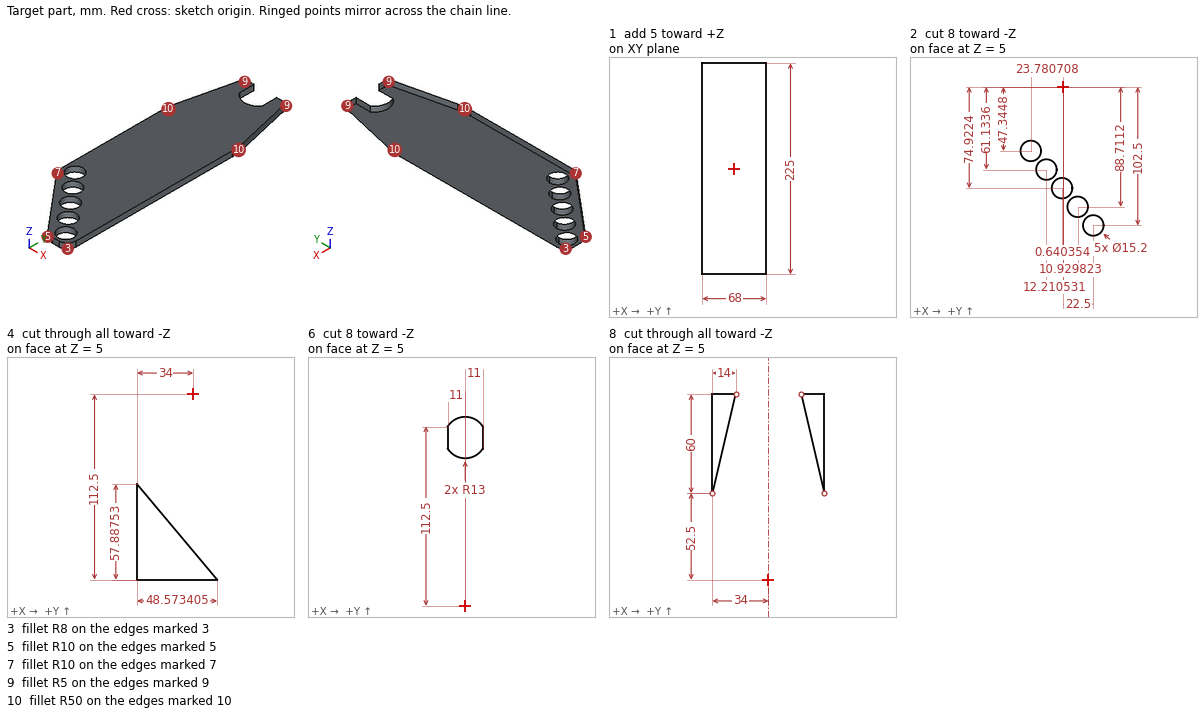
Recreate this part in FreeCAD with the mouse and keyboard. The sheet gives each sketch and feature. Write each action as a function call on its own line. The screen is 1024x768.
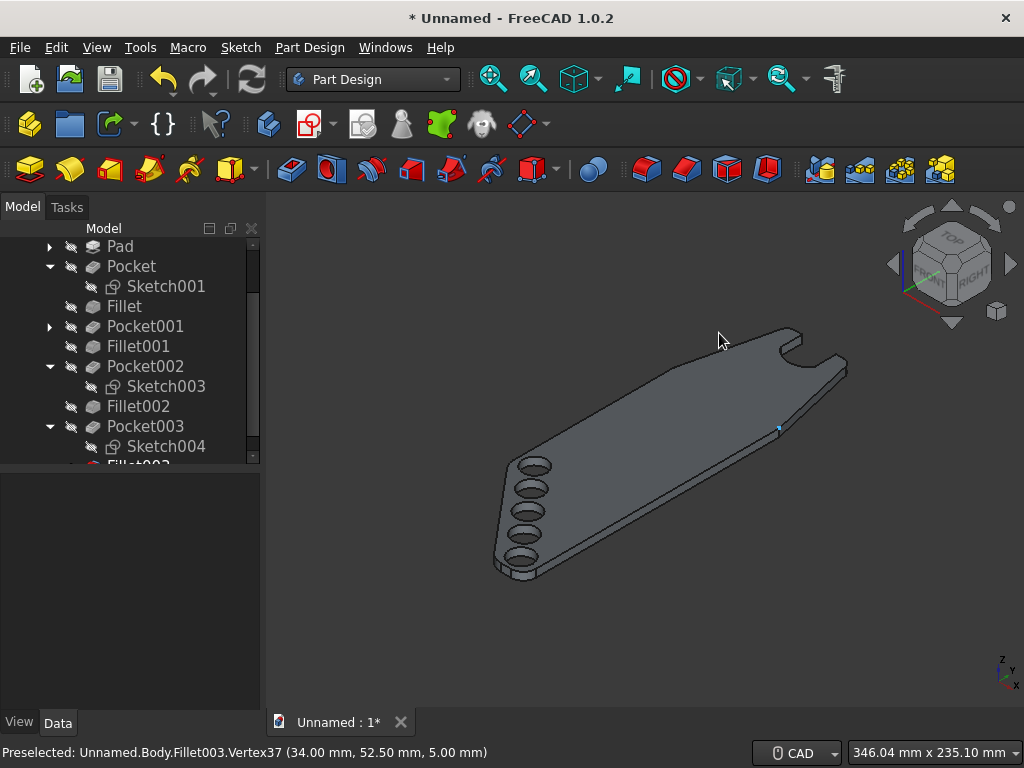
scroll(779, 432, up, 7)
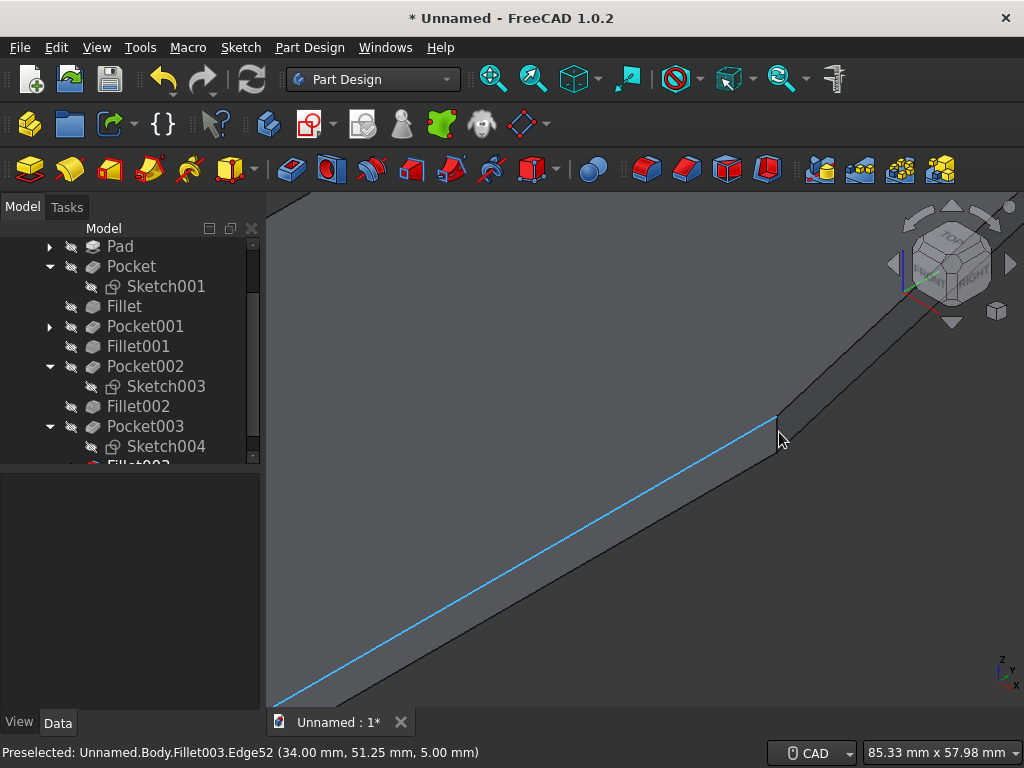
key(v)
key(f)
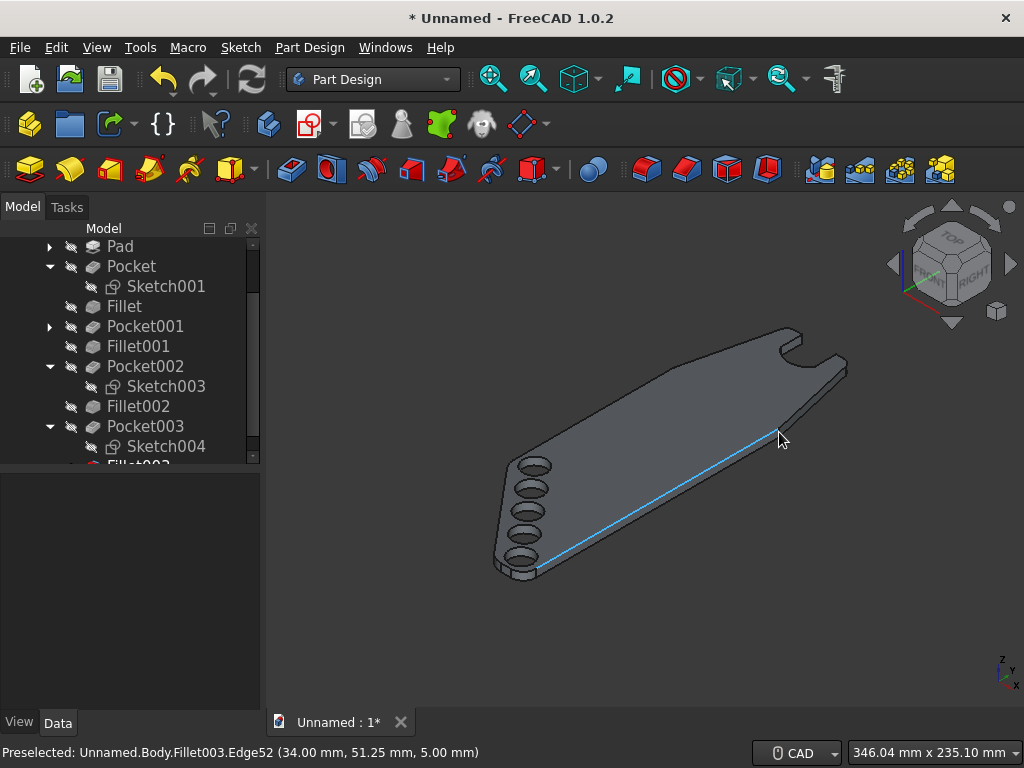
key(1)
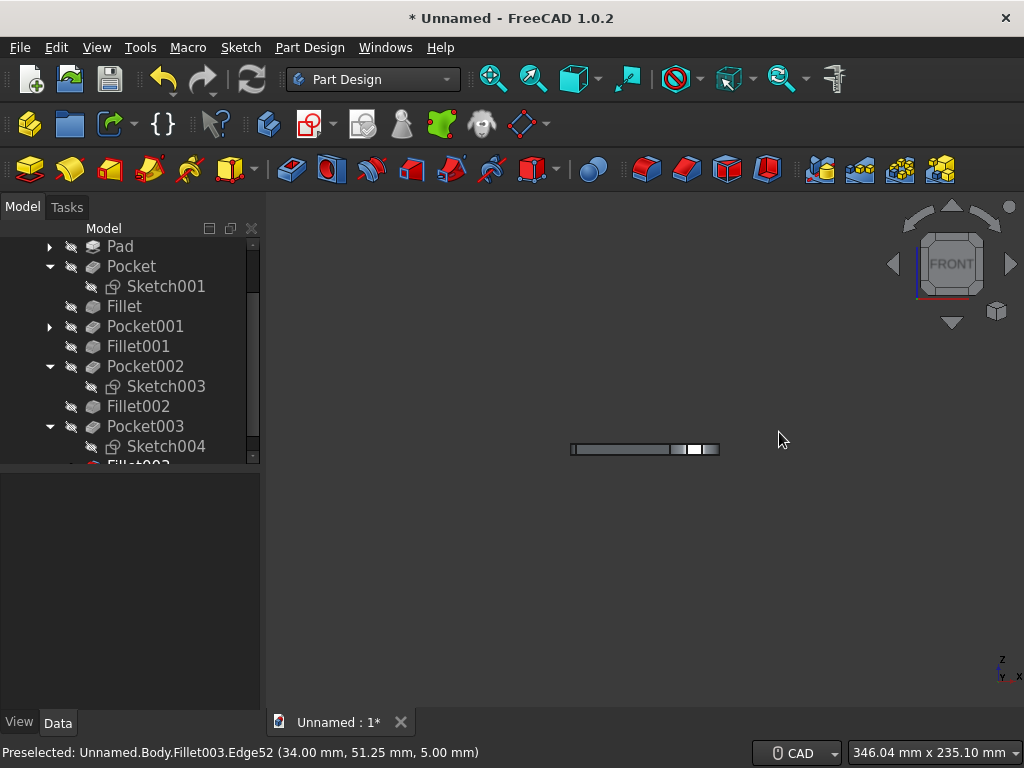
click(494, 80)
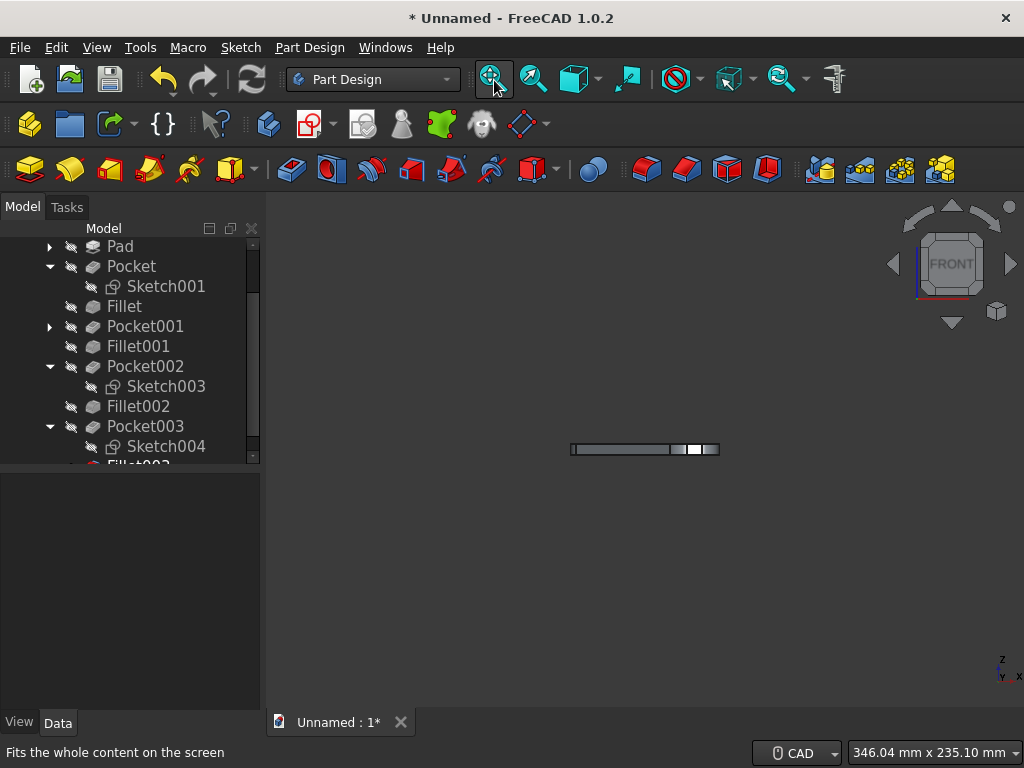
scroll(719, 449, up, 7)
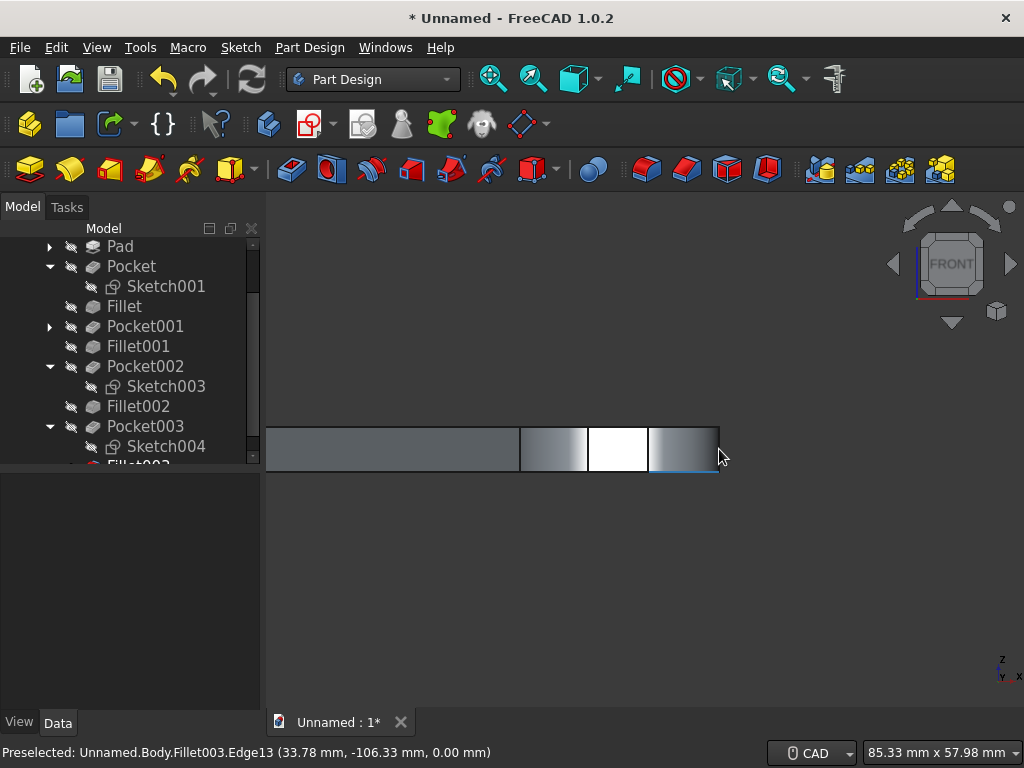
key(v)
key(f)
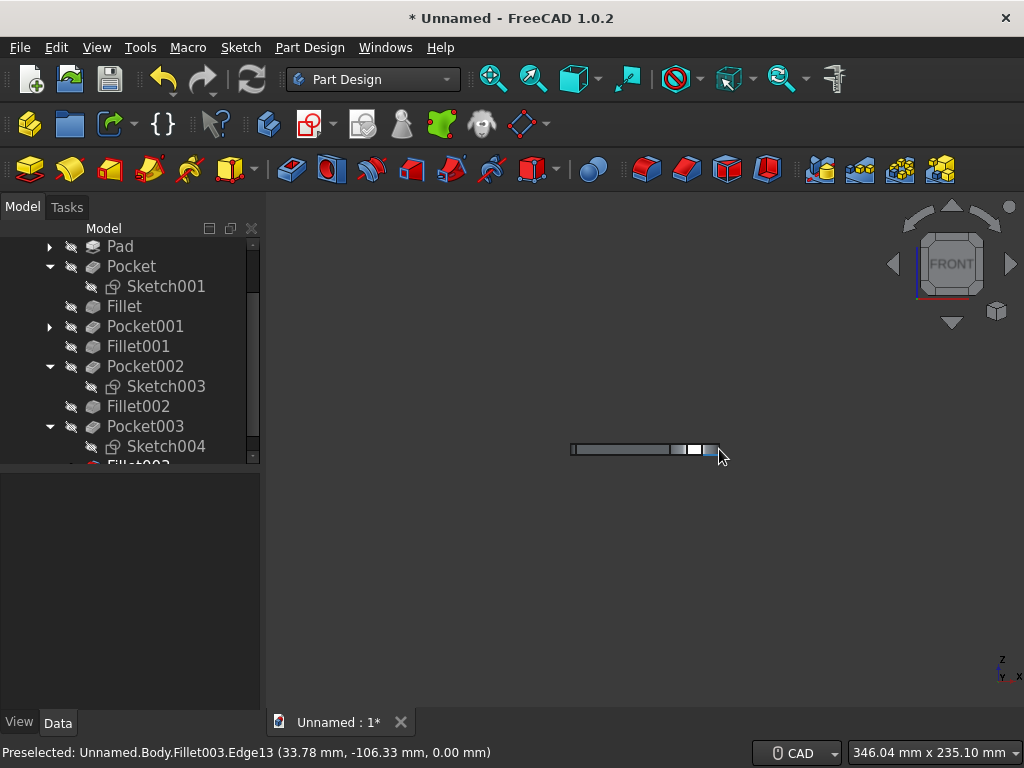
key(3)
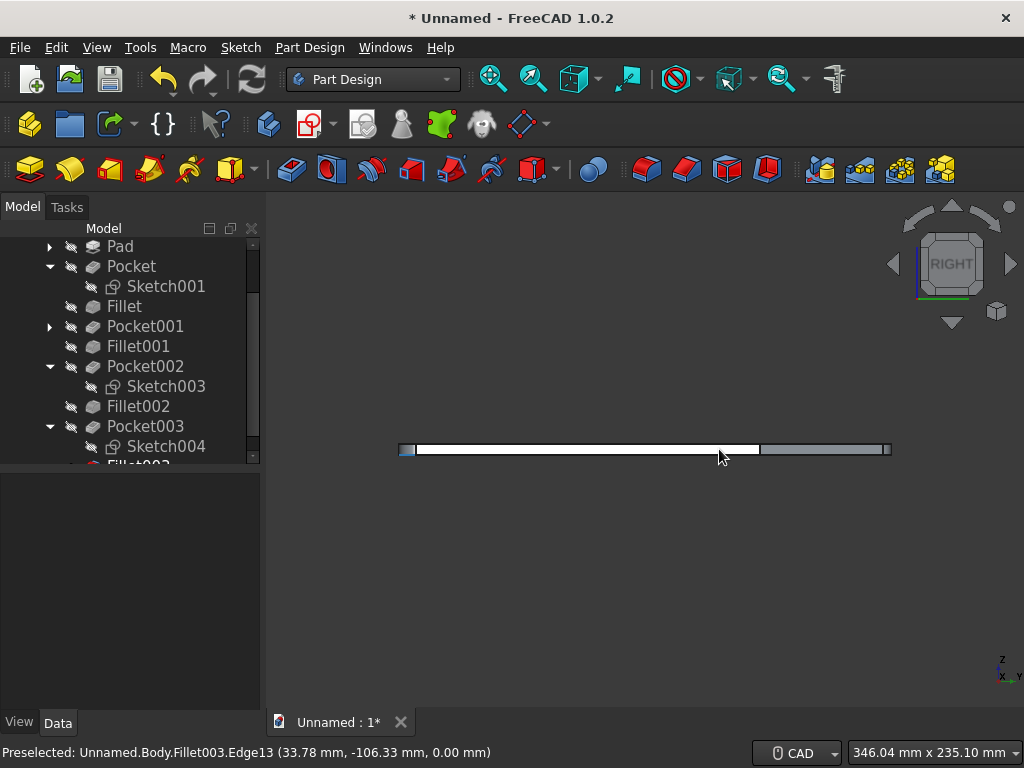
scroll(760, 448, up, 7)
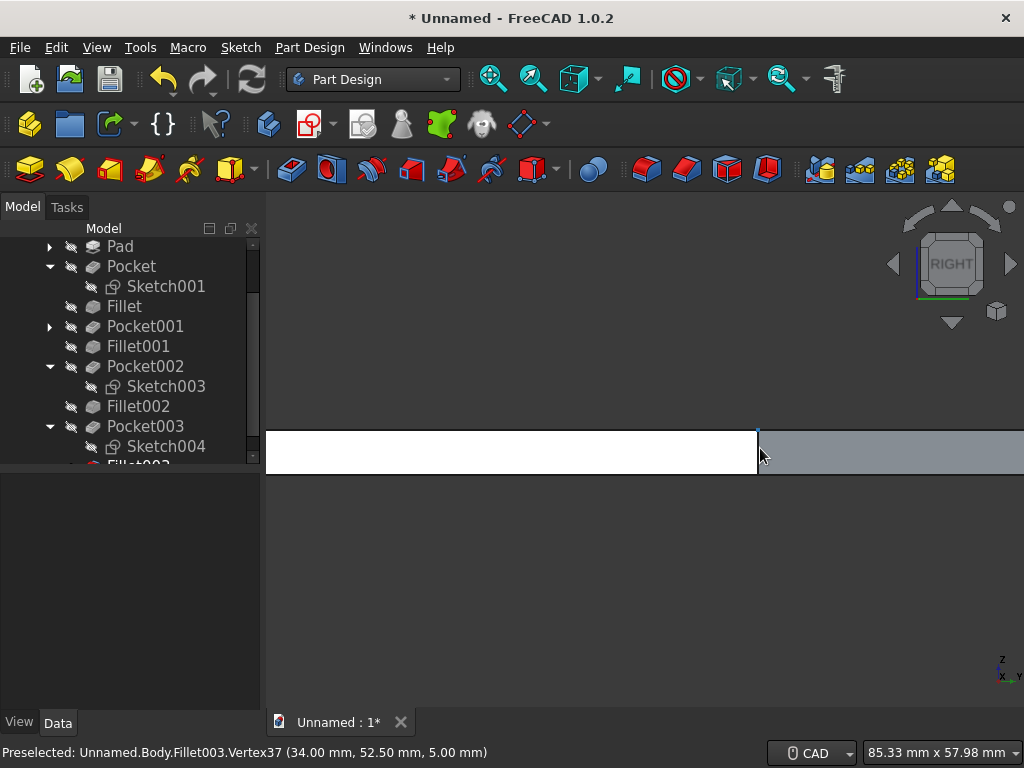
click(758, 452)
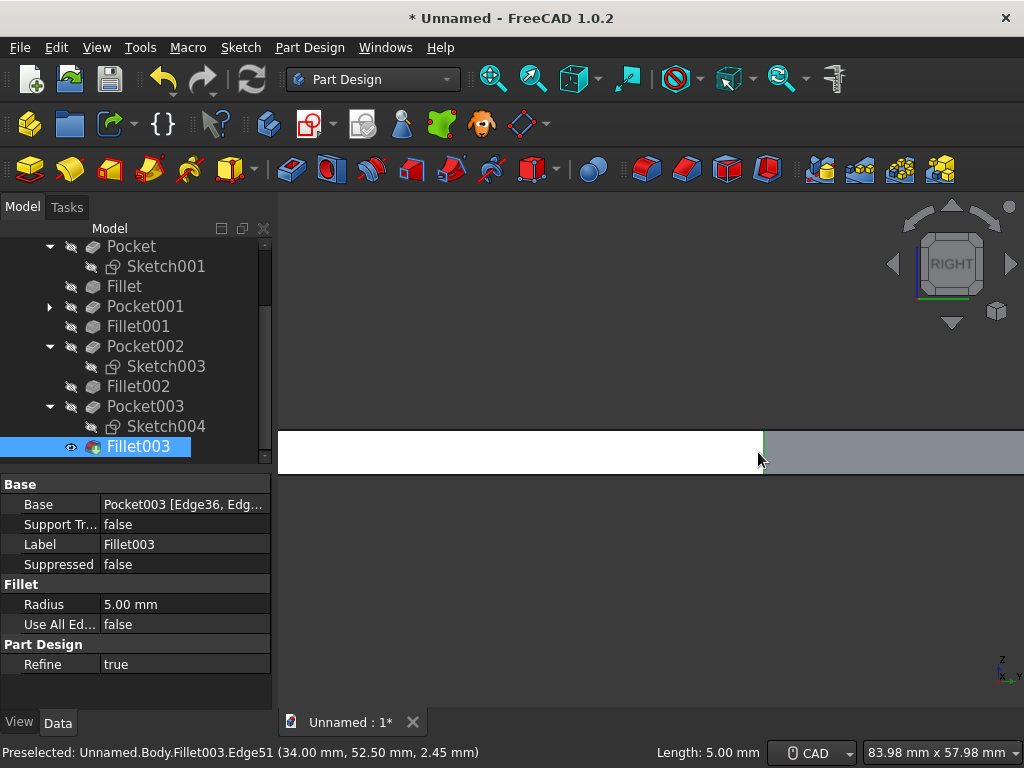
key(v)
key(f)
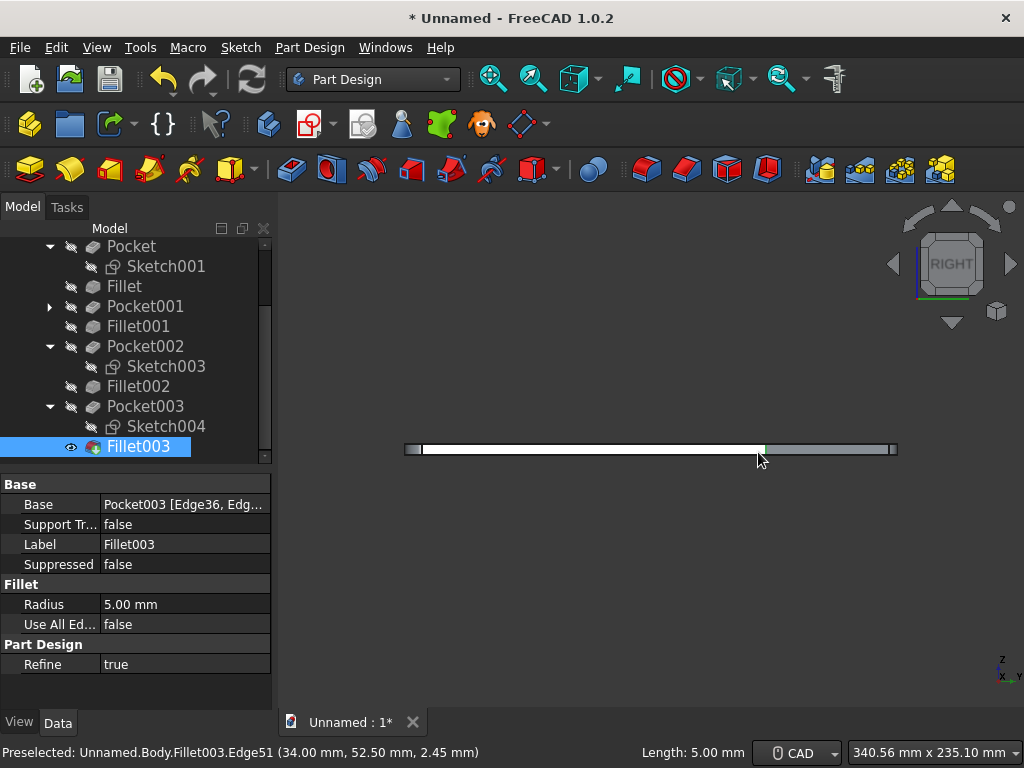
key(5)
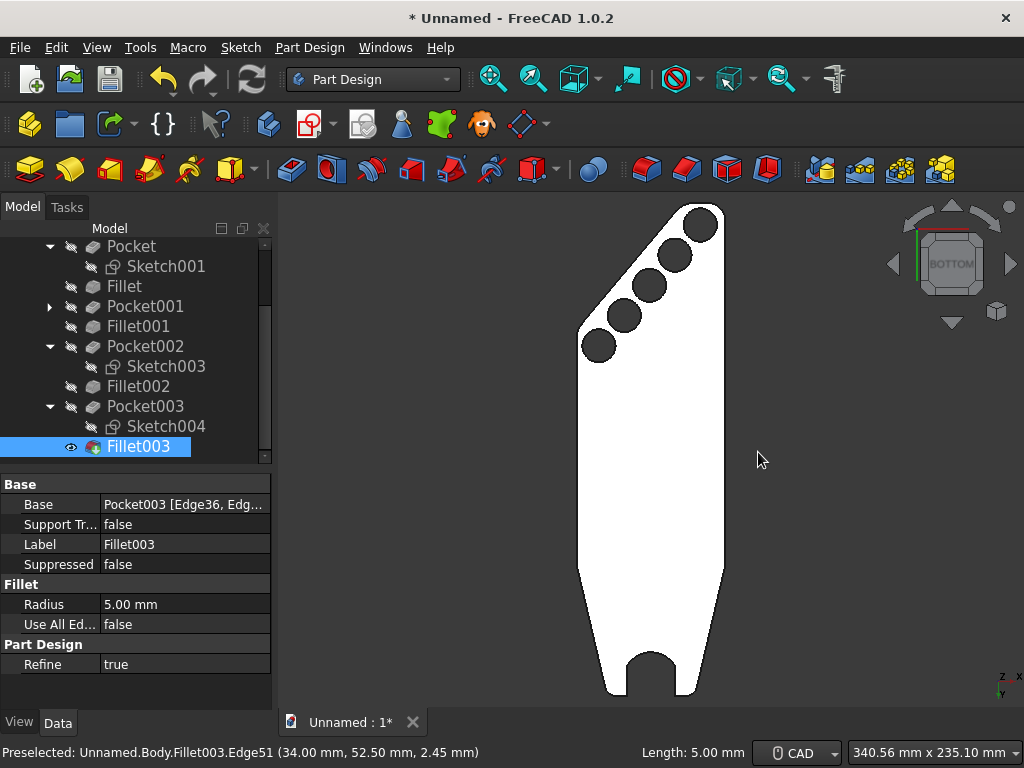
scroll(577, 564, up, 7)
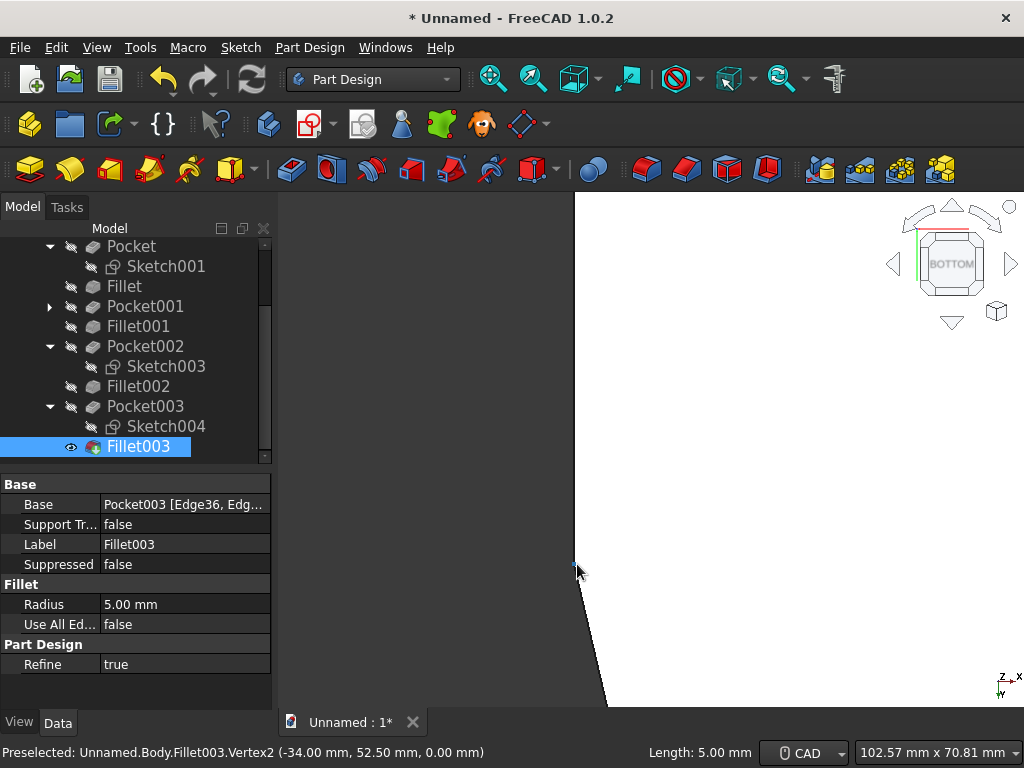
click(494, 80)